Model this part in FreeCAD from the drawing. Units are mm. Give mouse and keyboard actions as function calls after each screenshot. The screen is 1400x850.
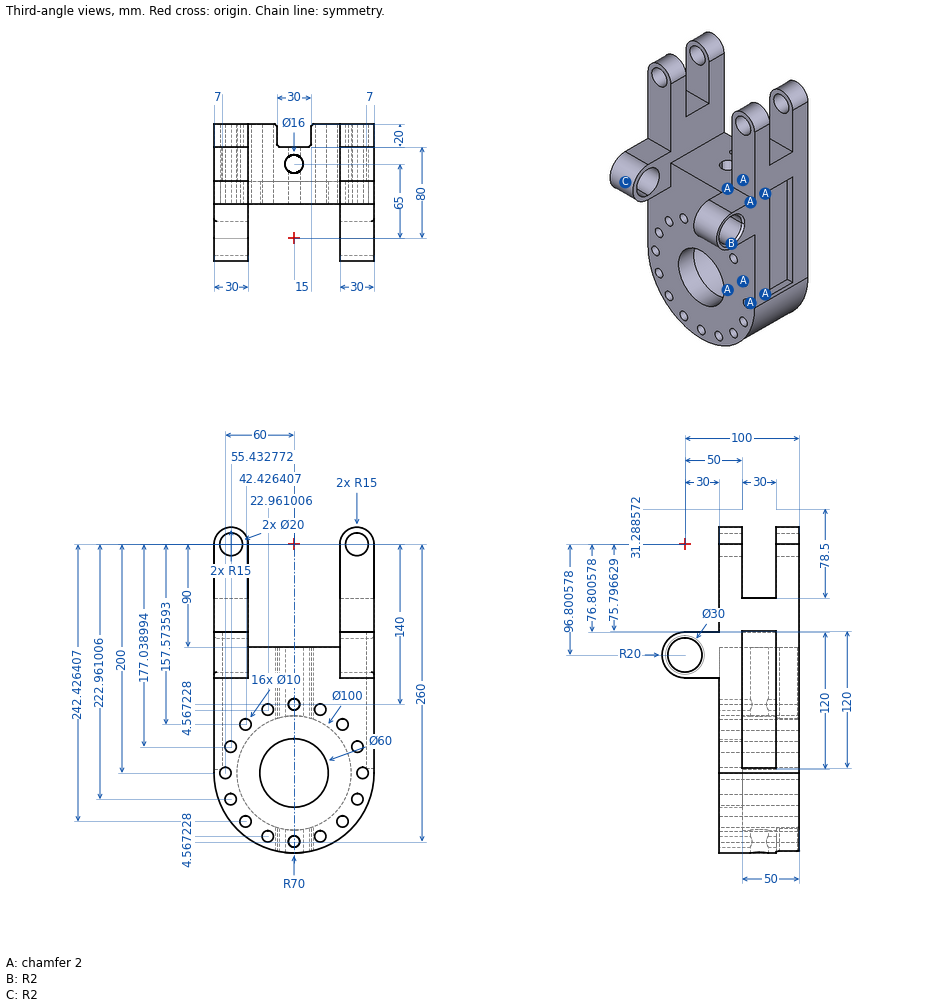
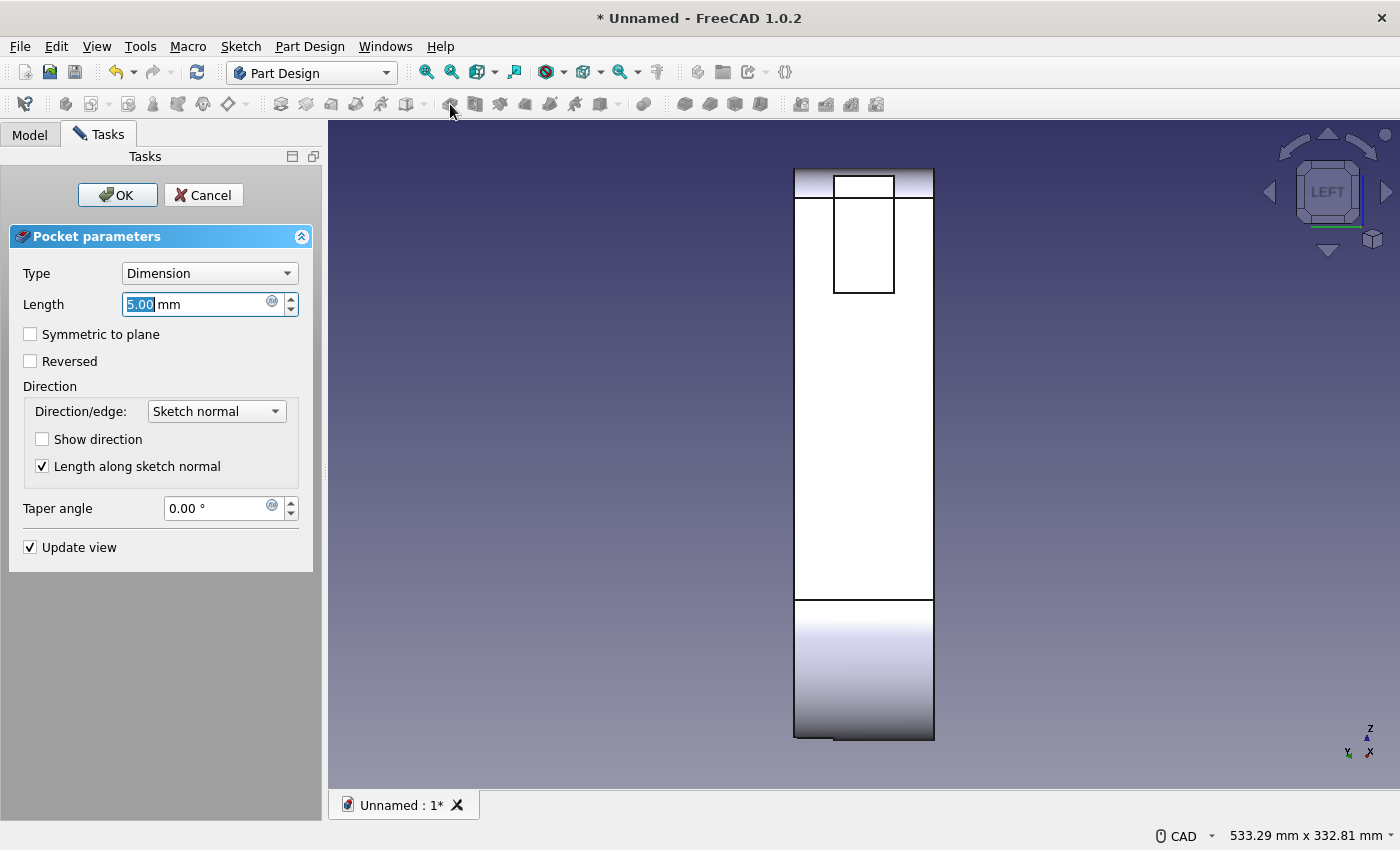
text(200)
key(Tab)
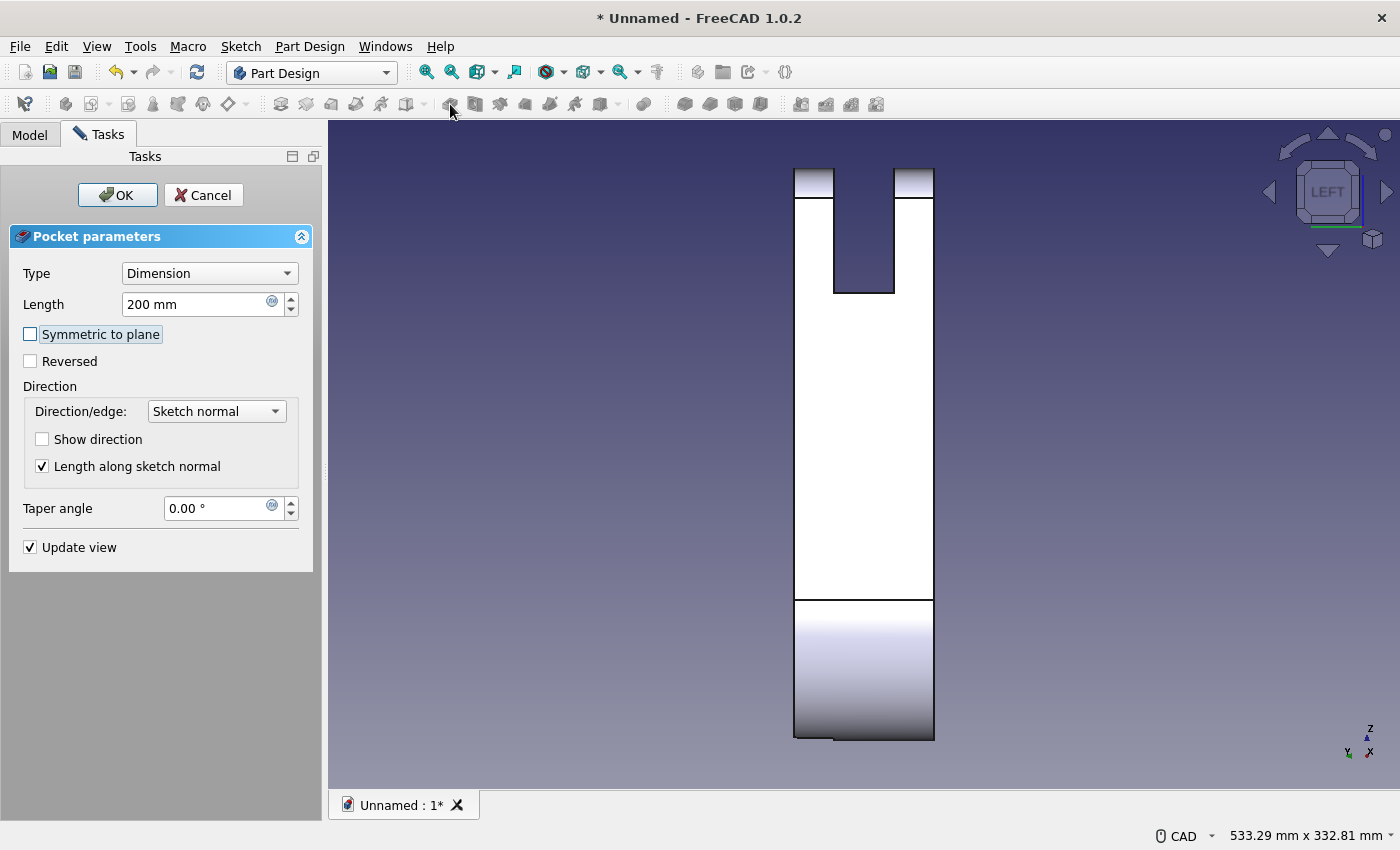
click(118, 195)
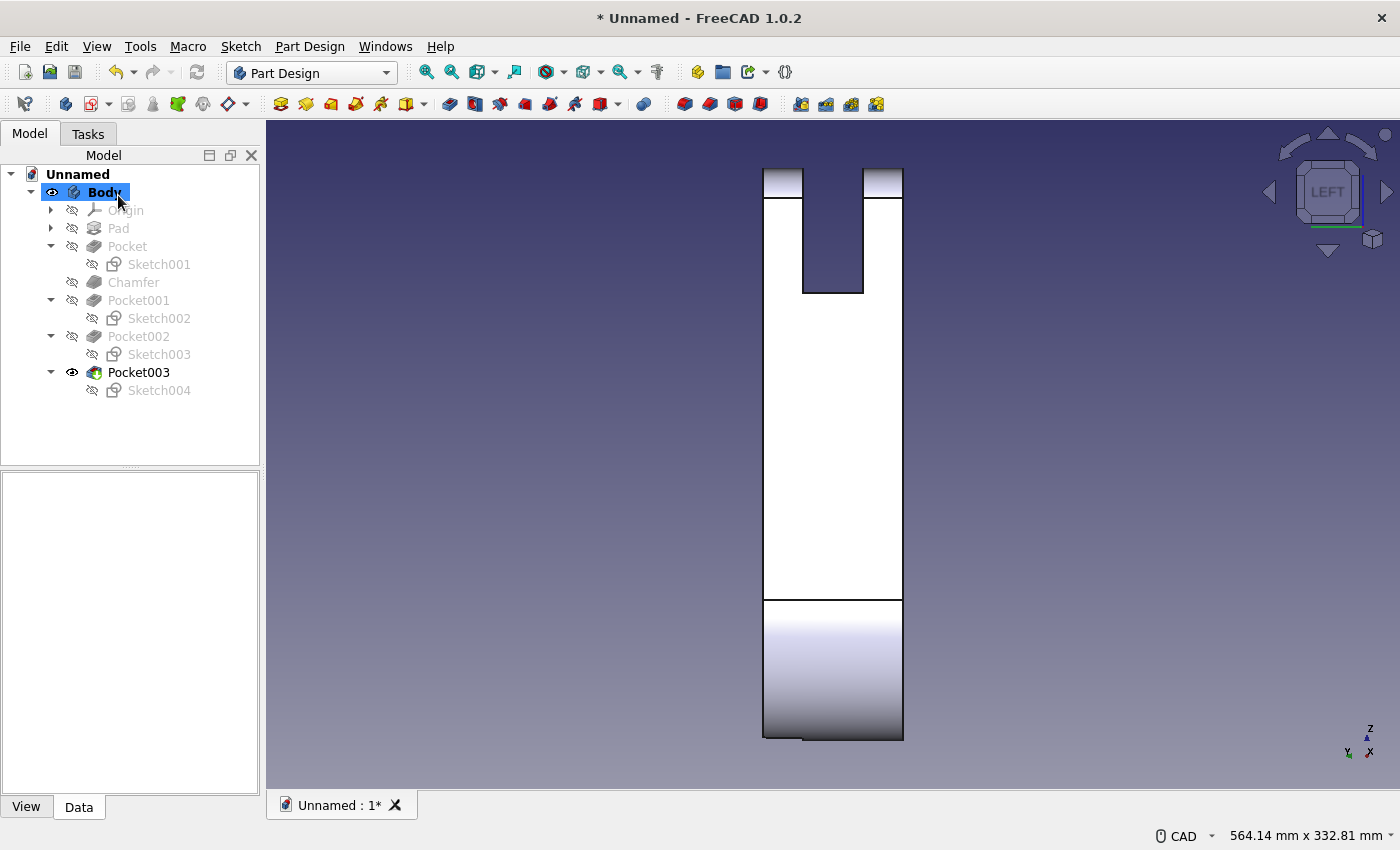
key(0)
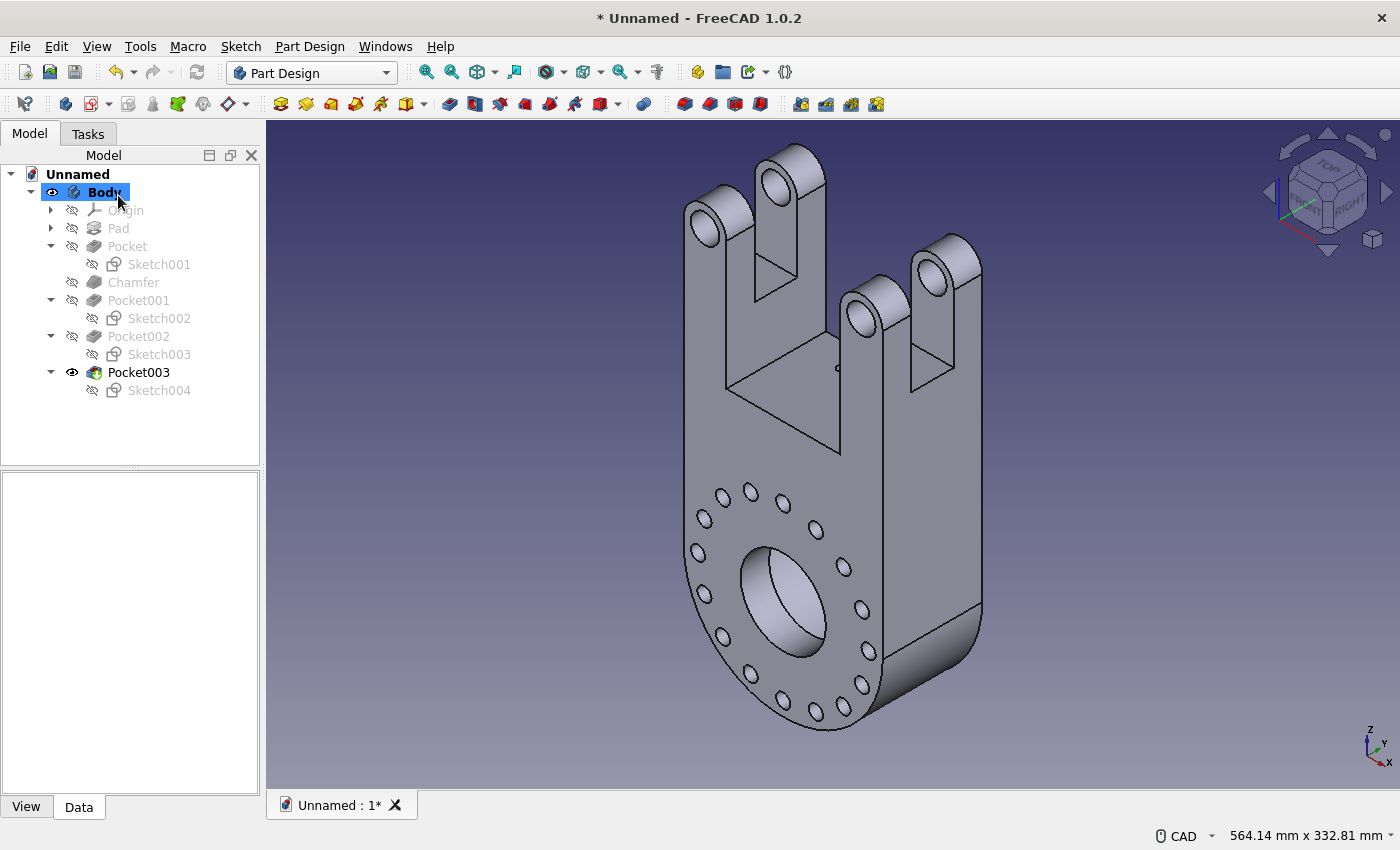
click(819, 400)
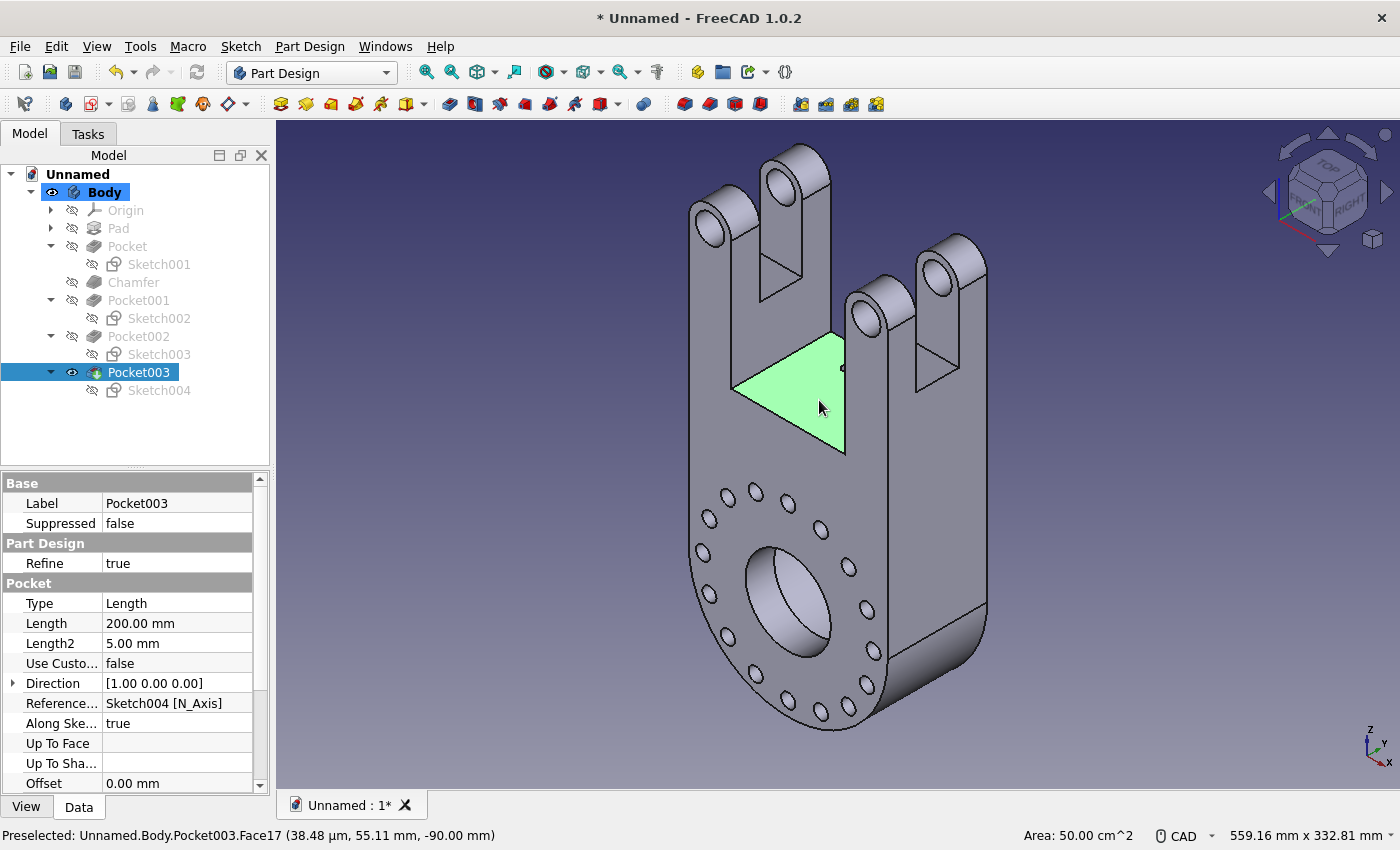
click(90, 104)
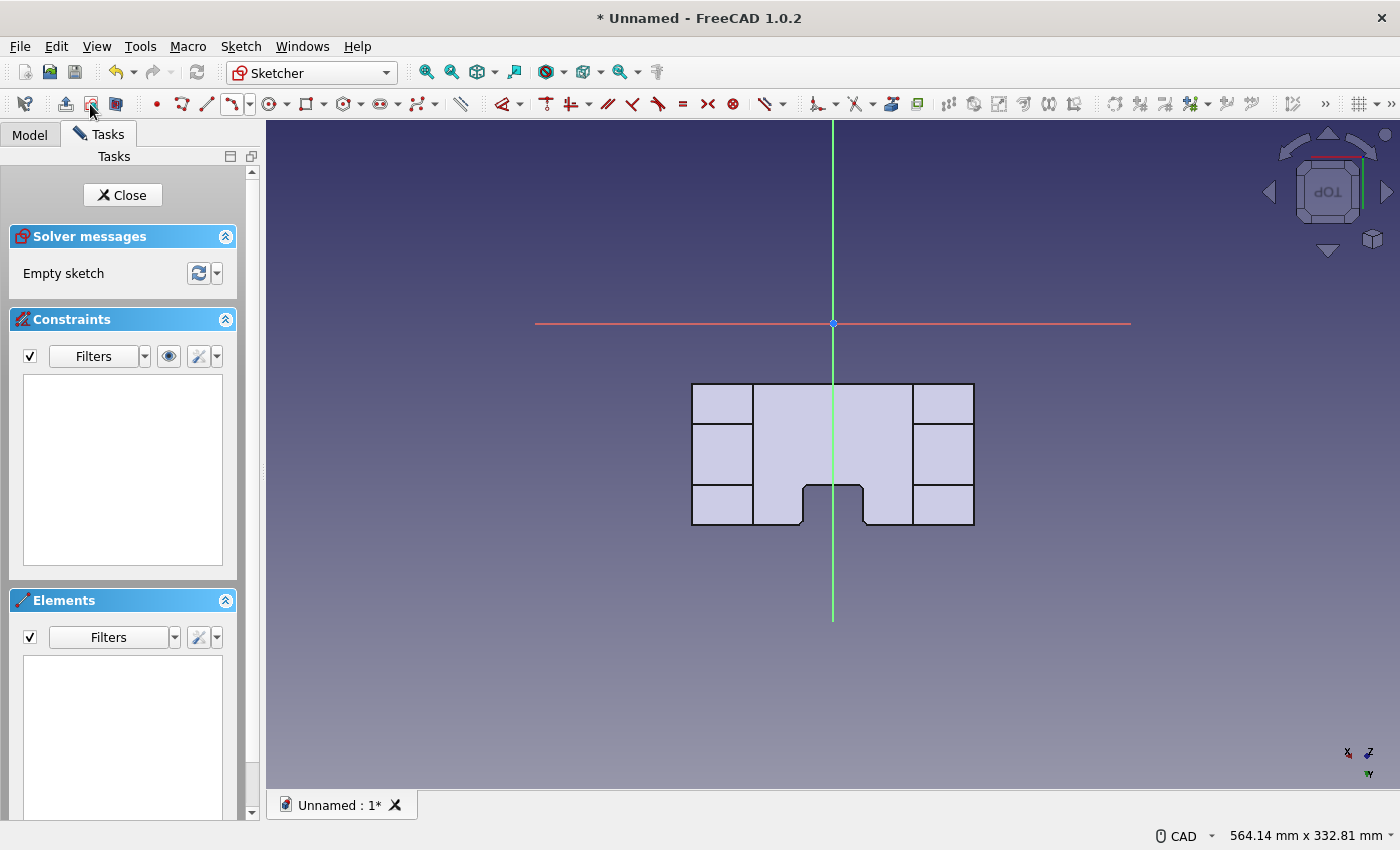
key(q)
key(s)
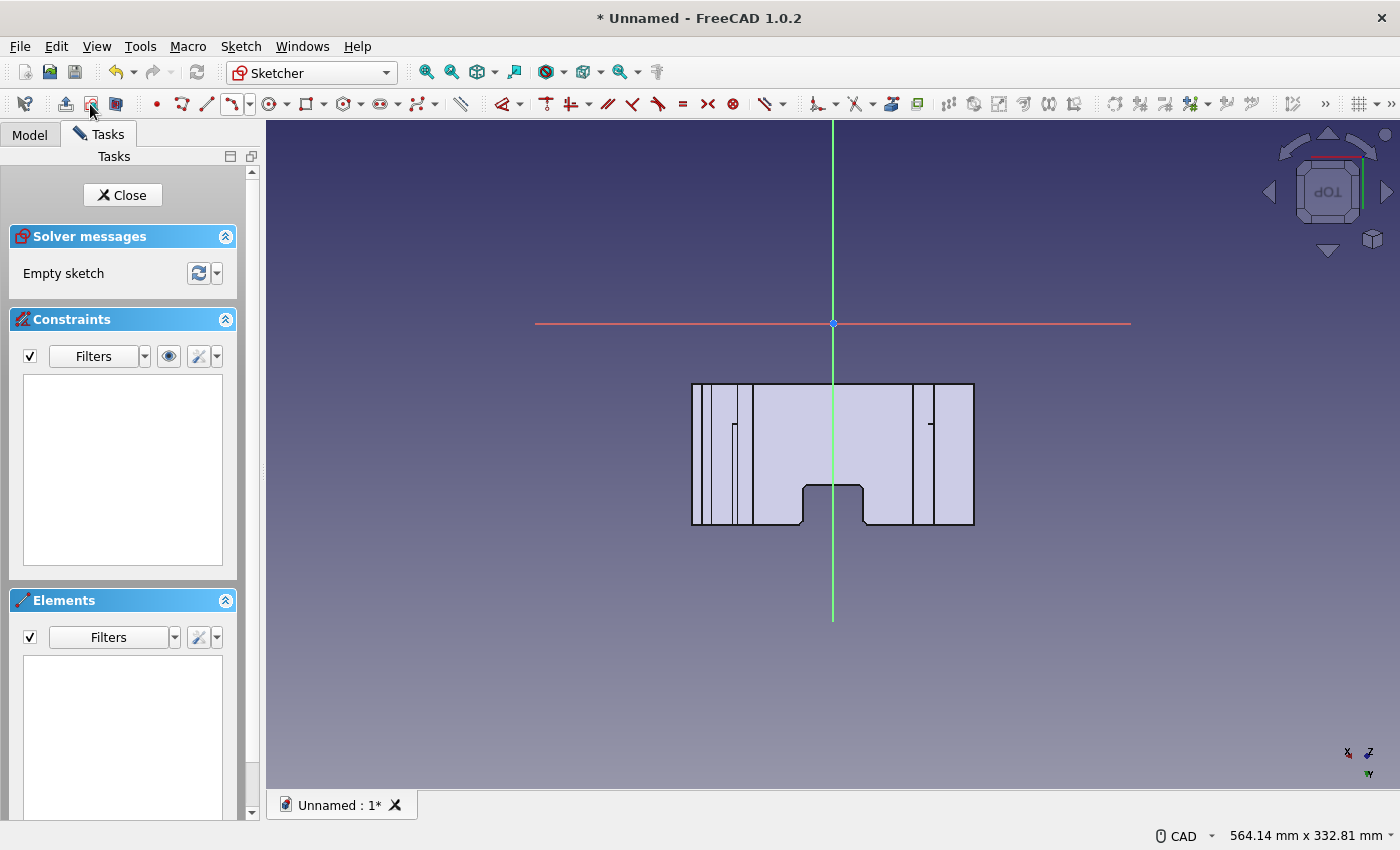
scroll(838, 454, up, 13)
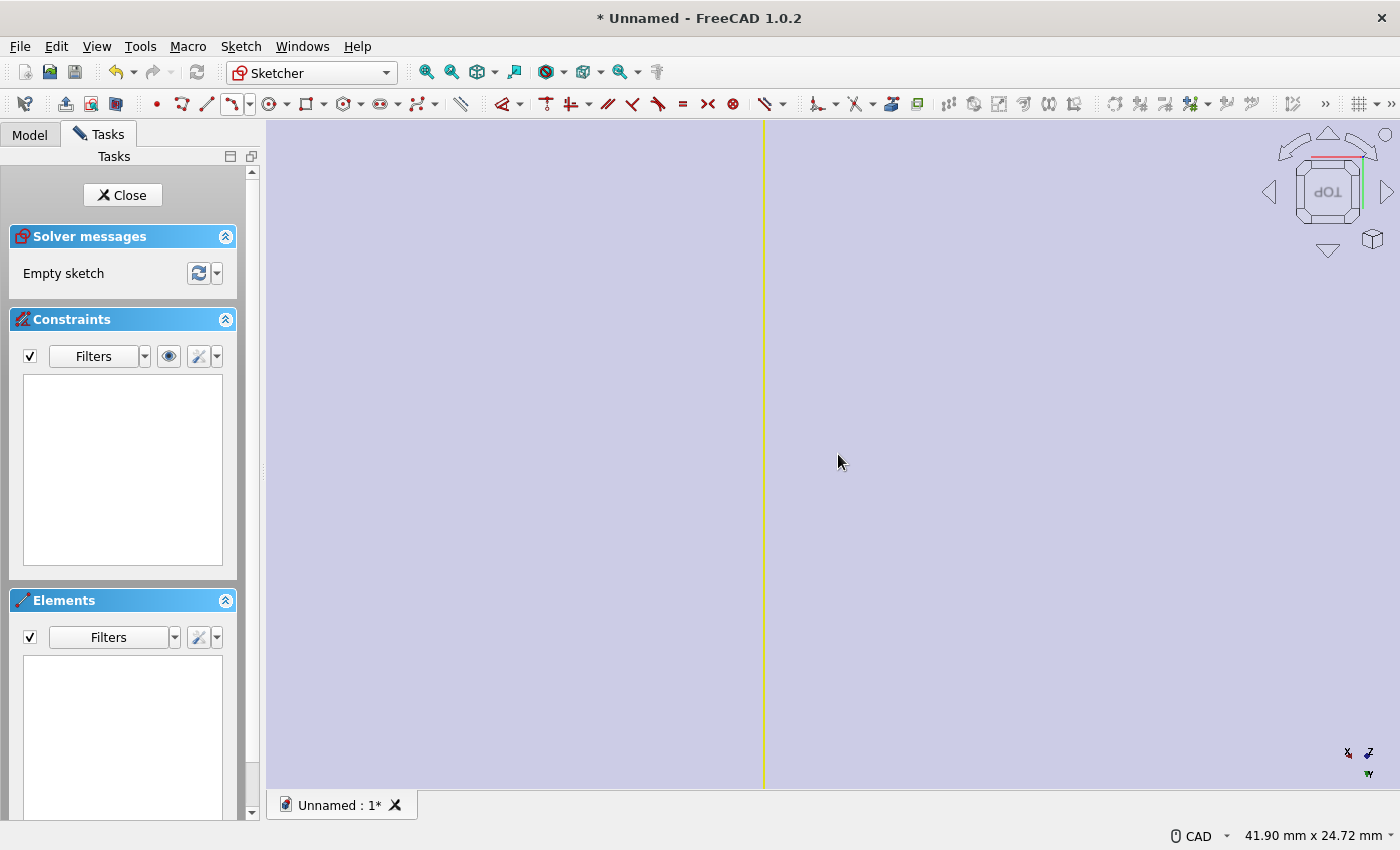
click(268, 104)